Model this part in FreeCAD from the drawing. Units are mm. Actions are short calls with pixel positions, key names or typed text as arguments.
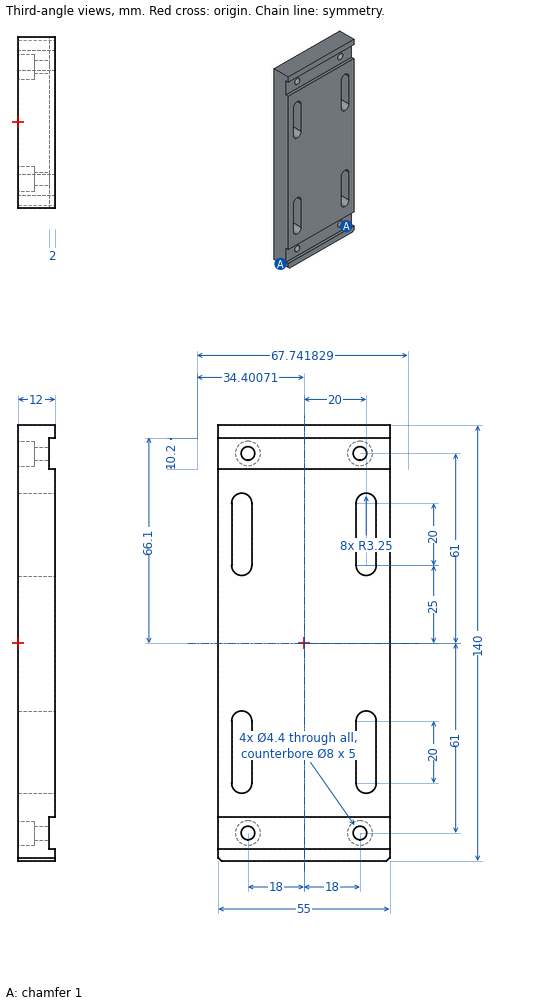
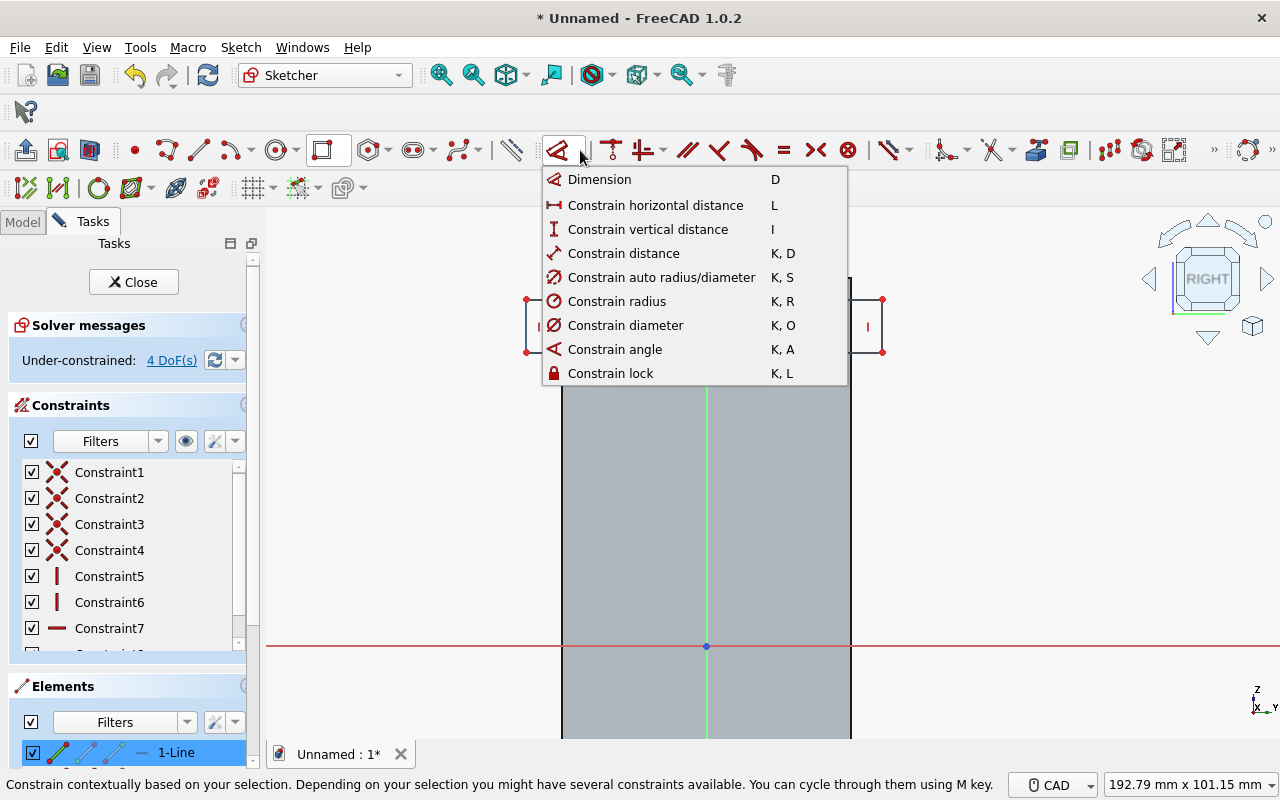
click(695, 229)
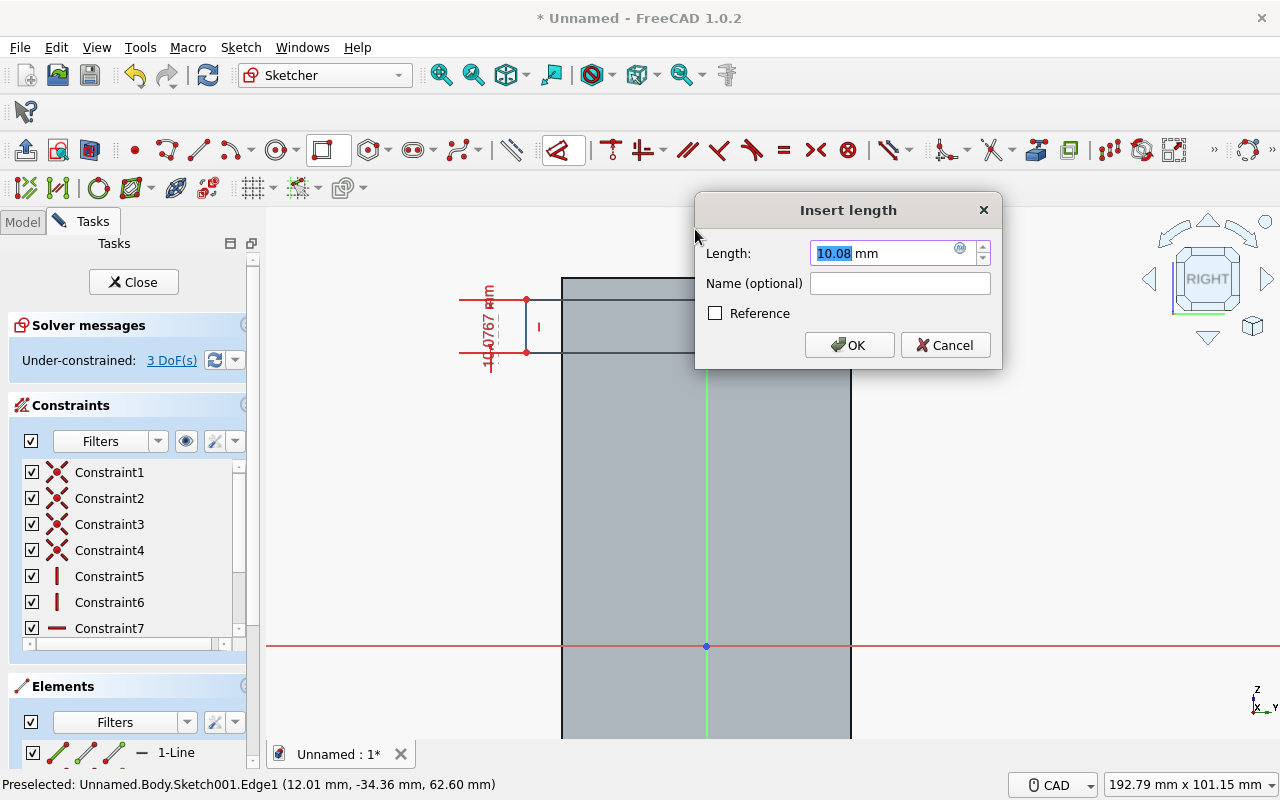
text(10.2)
key(Return)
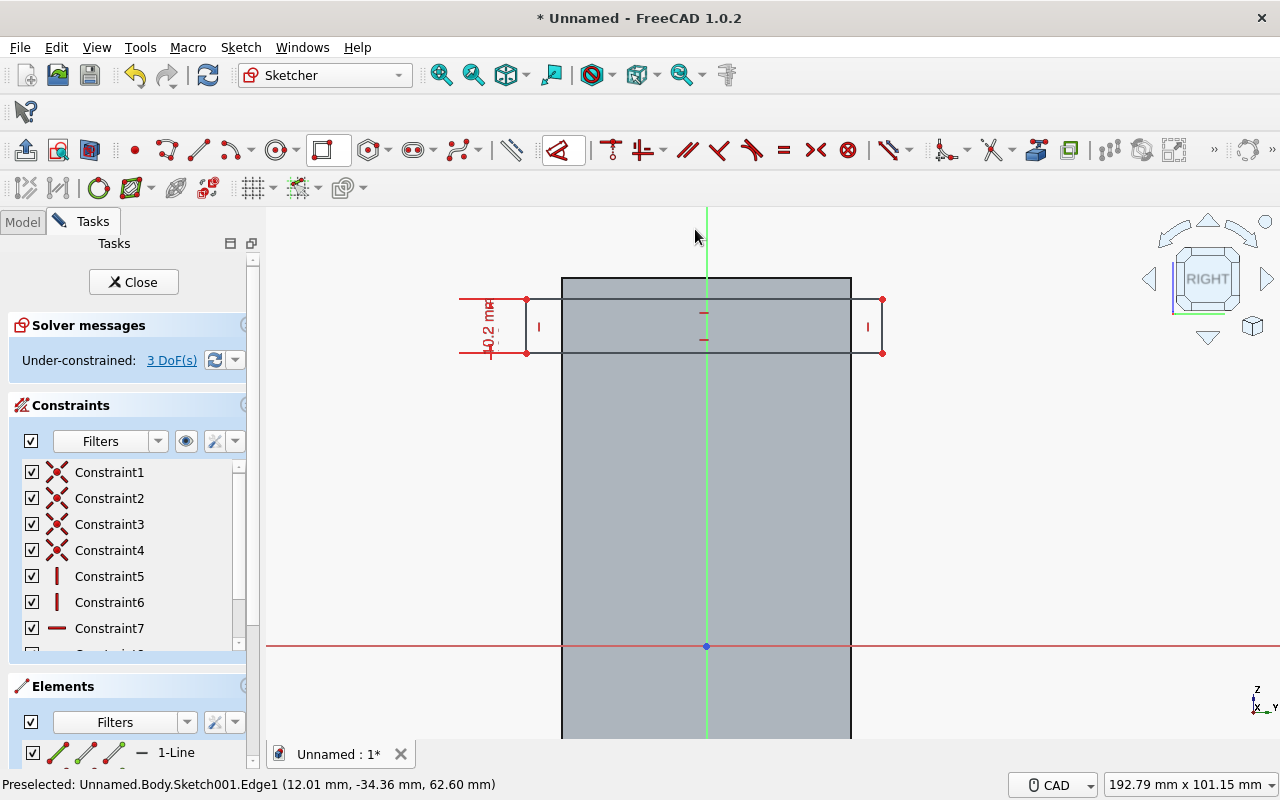
click(526, 299)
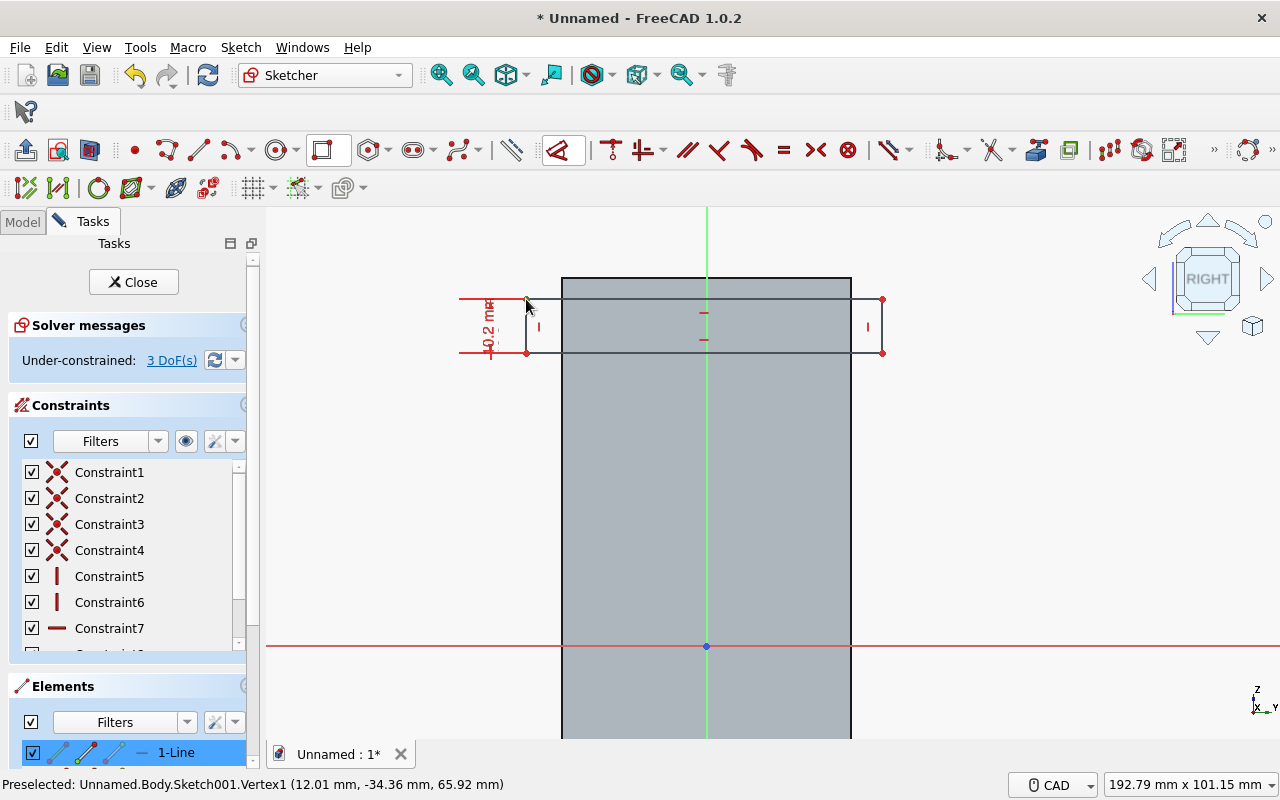
key(i)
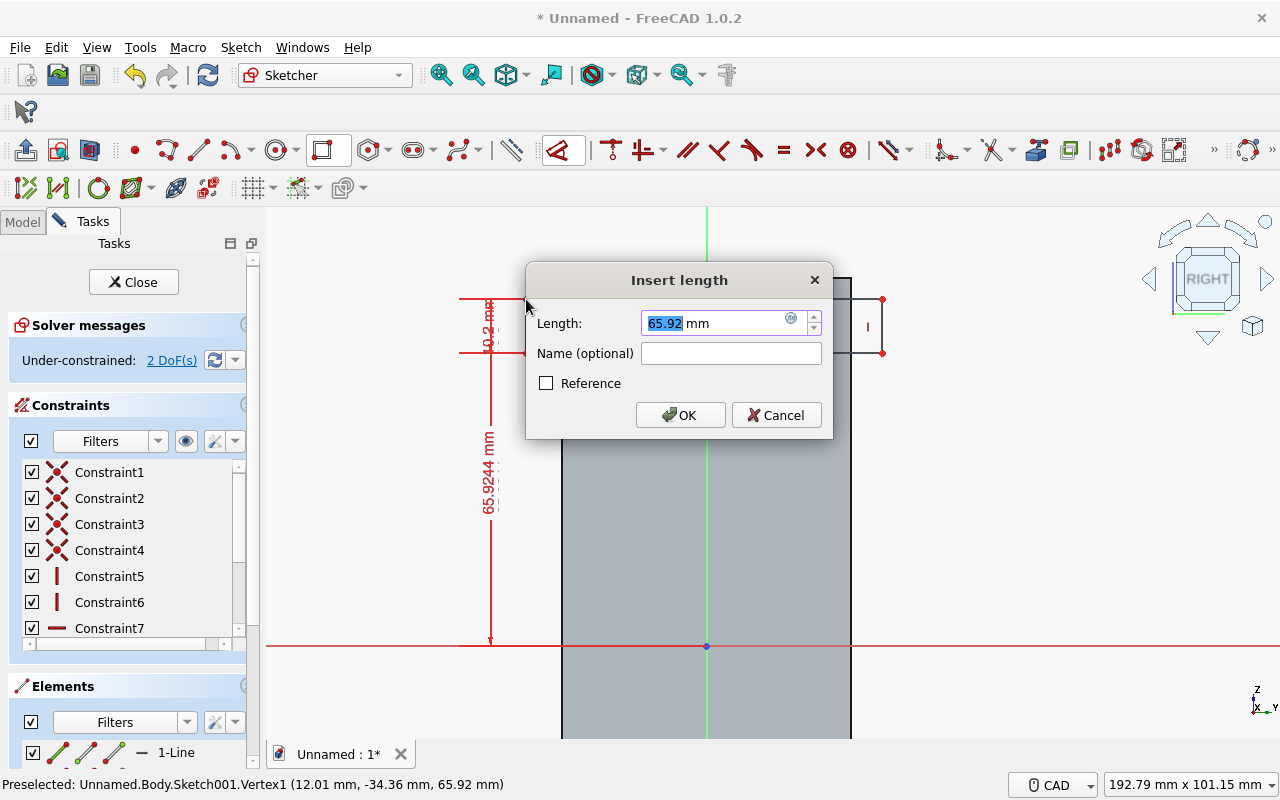
text(66.1)
key(Return)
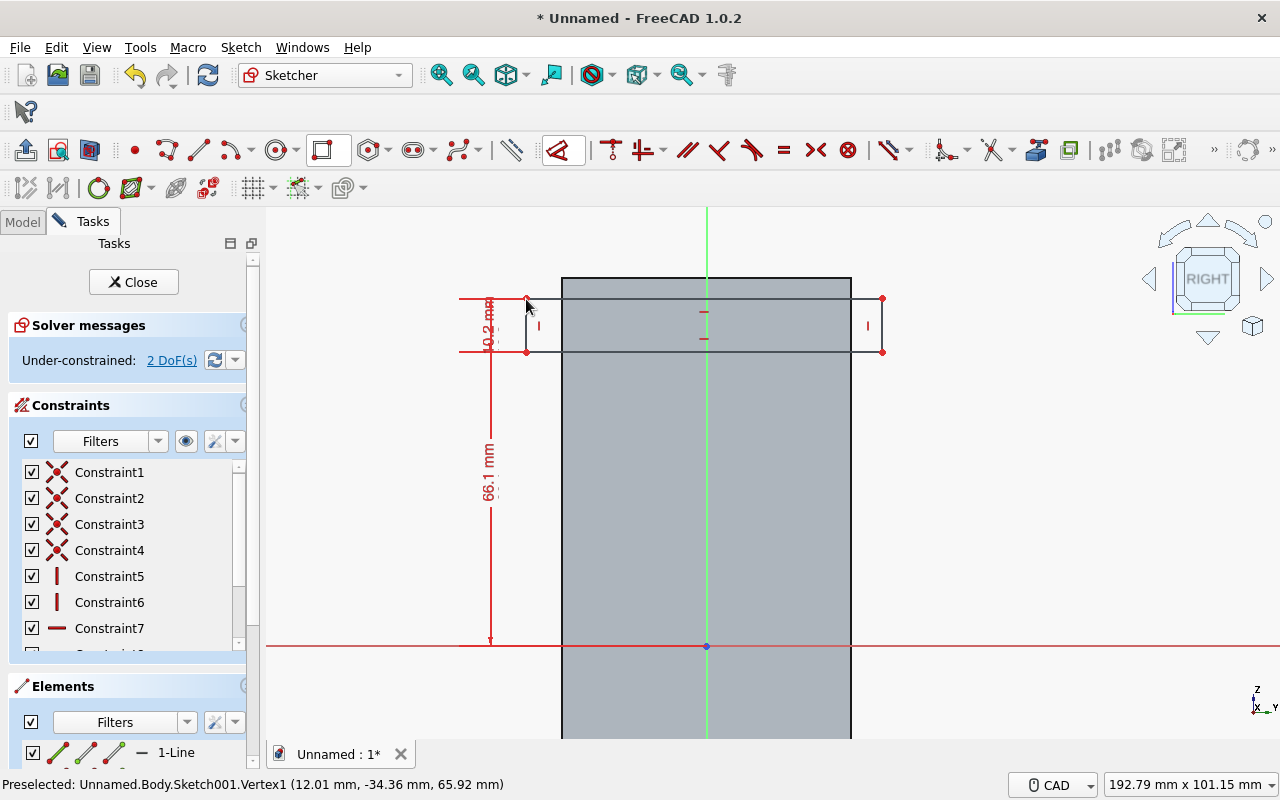
click(633, 352)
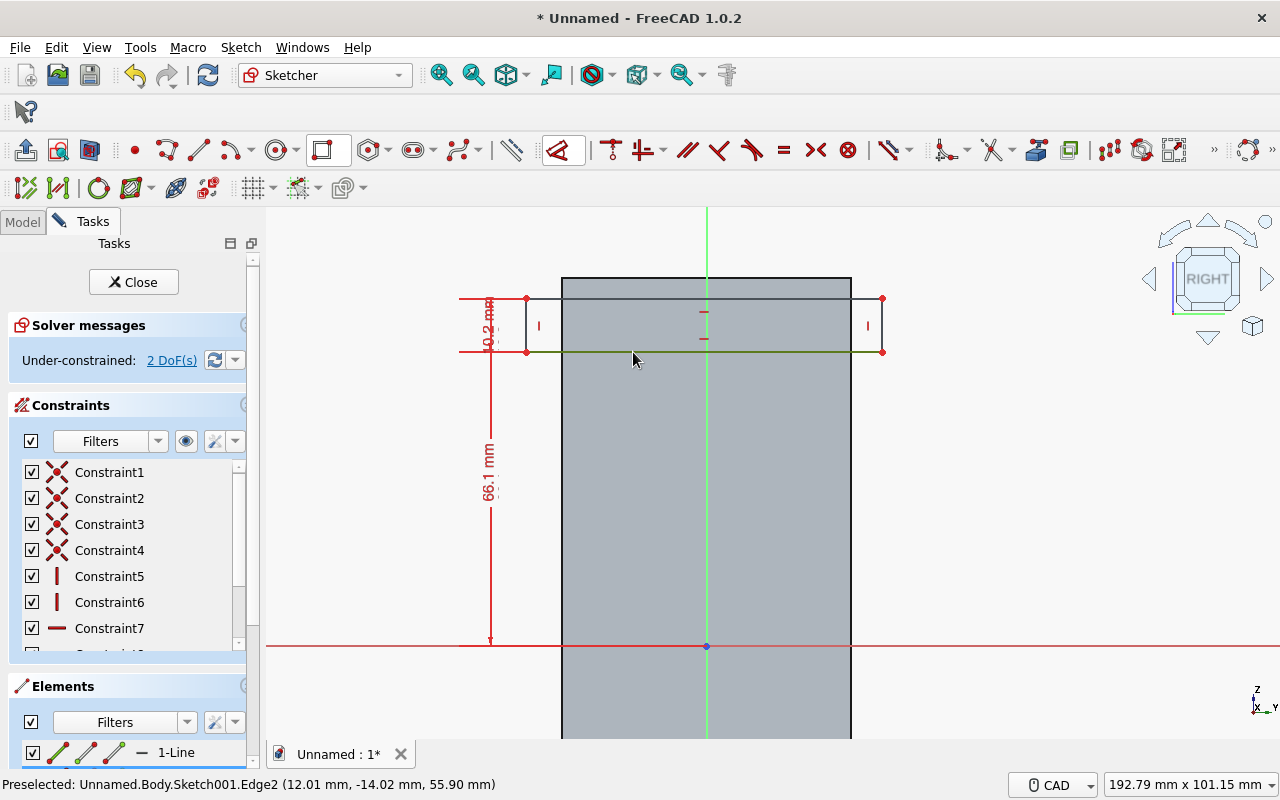
click(580, 150)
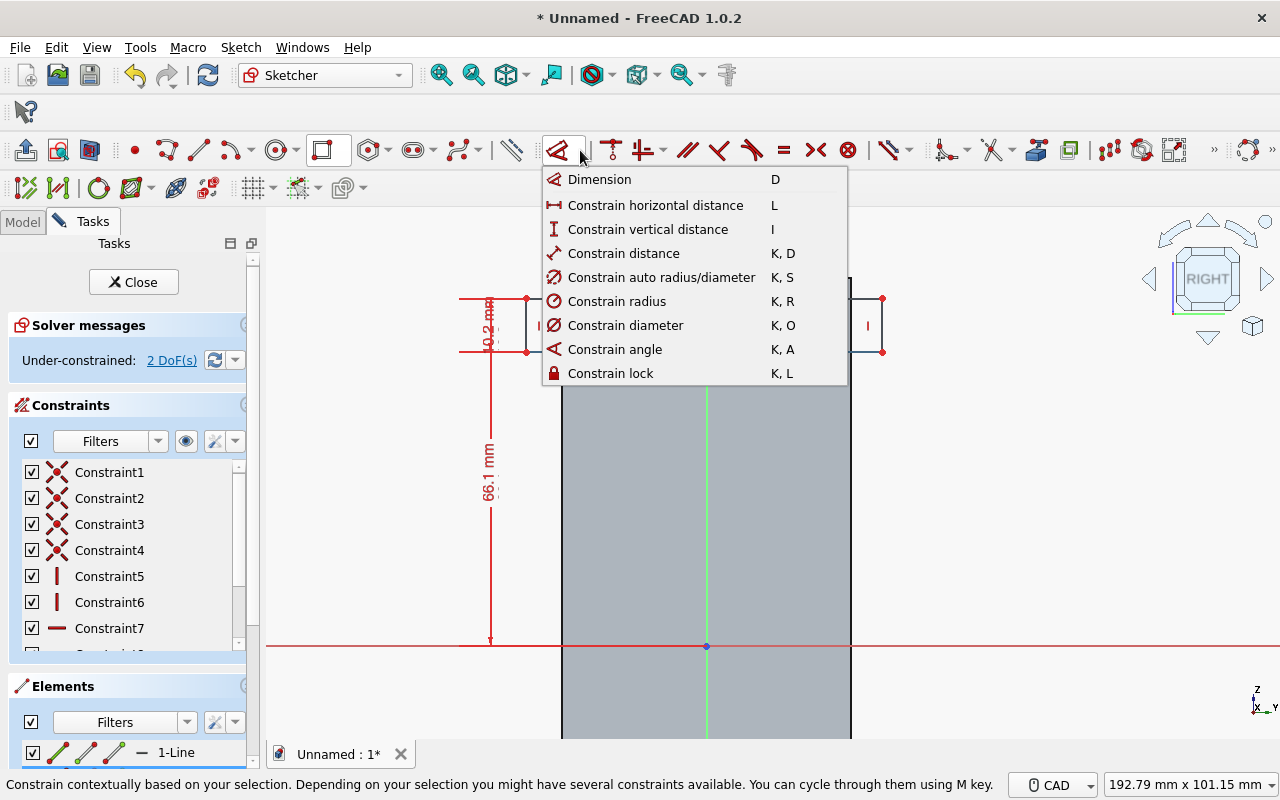
click(695, 205)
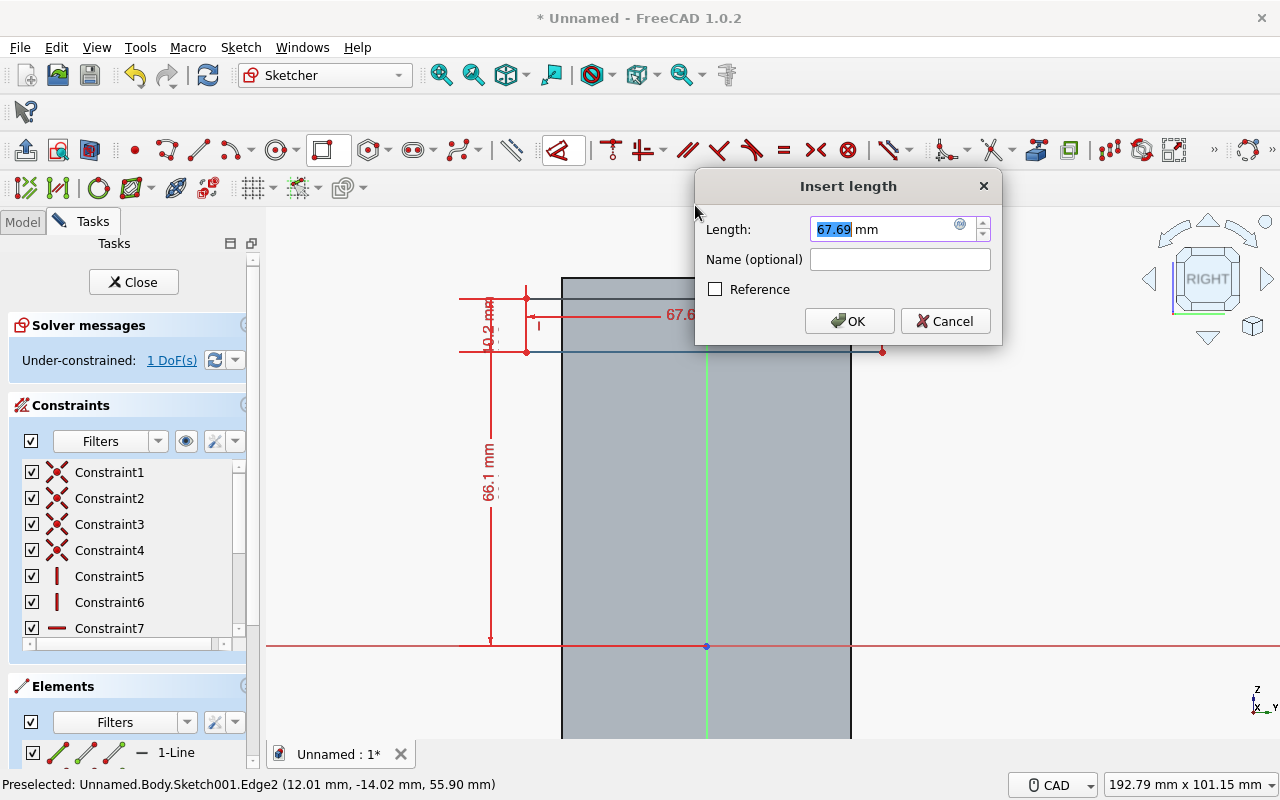
text(67.741829)
key(Return)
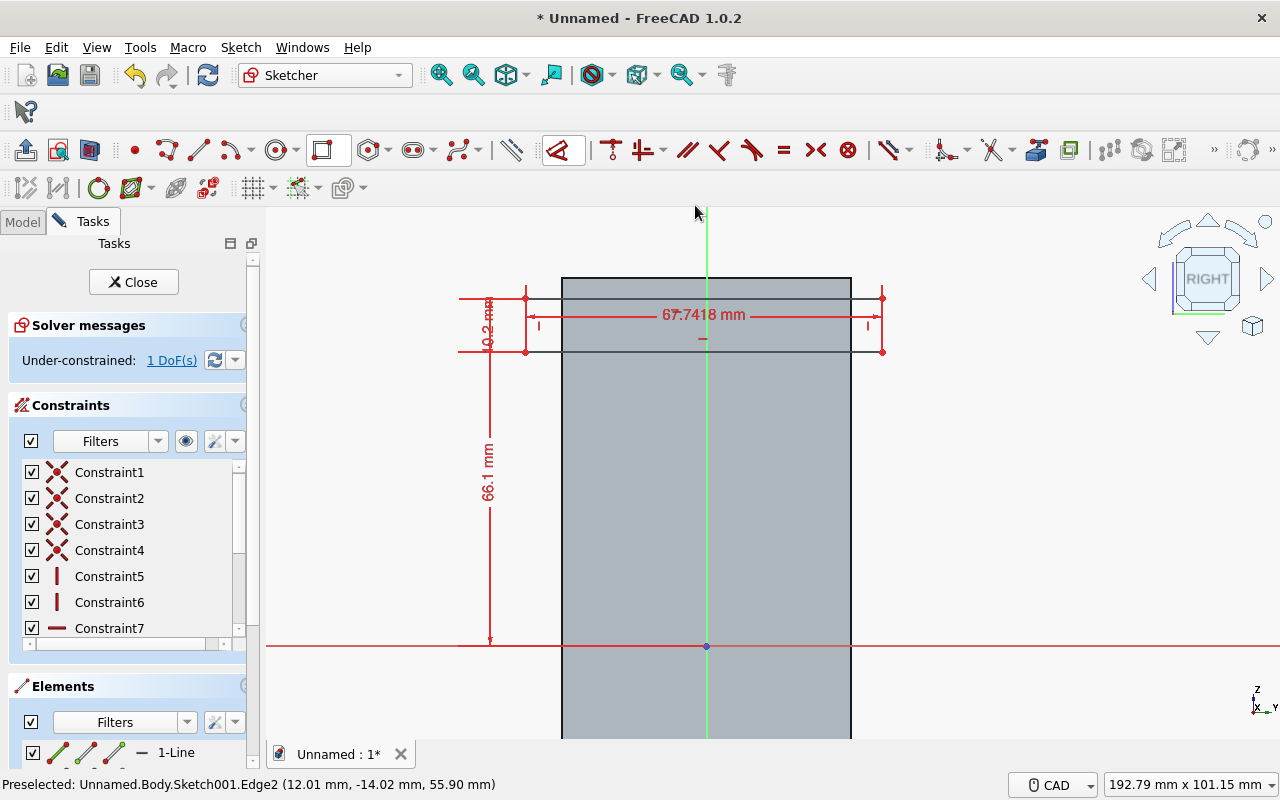
click(526, 299)